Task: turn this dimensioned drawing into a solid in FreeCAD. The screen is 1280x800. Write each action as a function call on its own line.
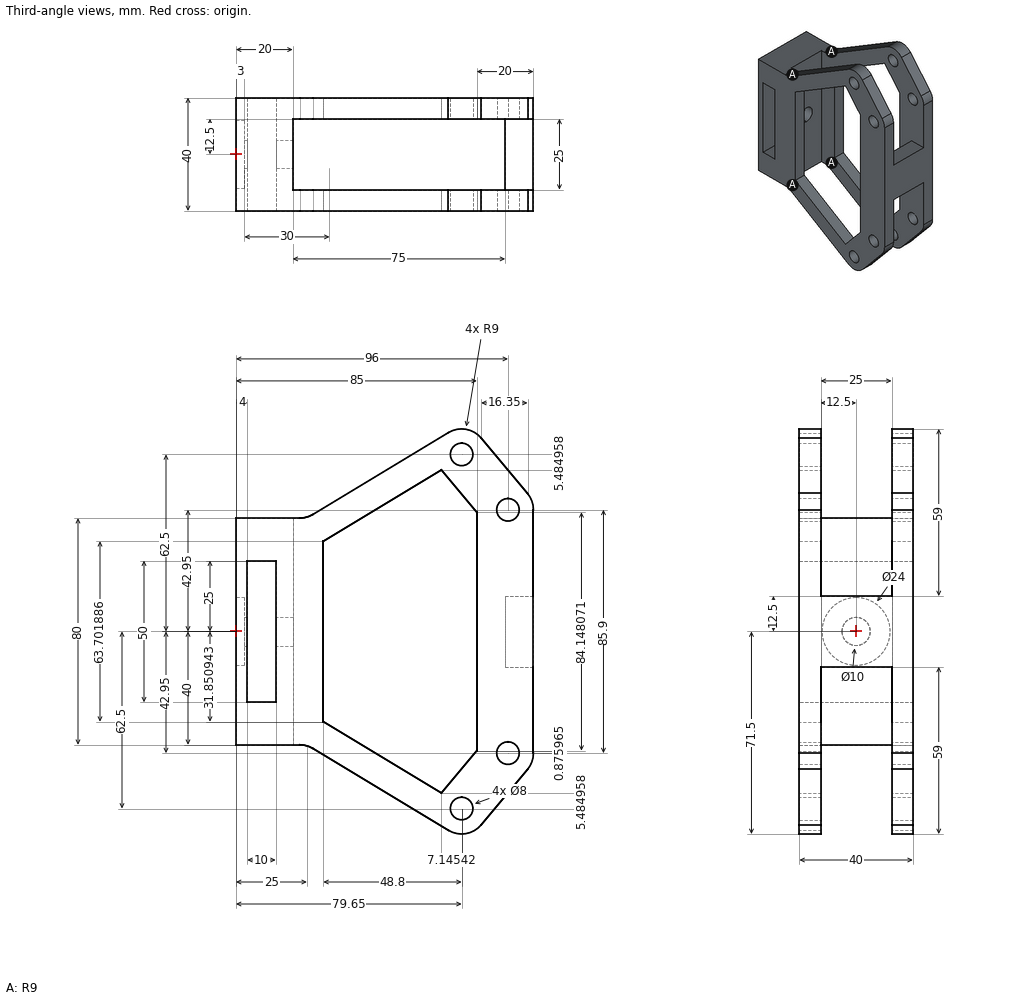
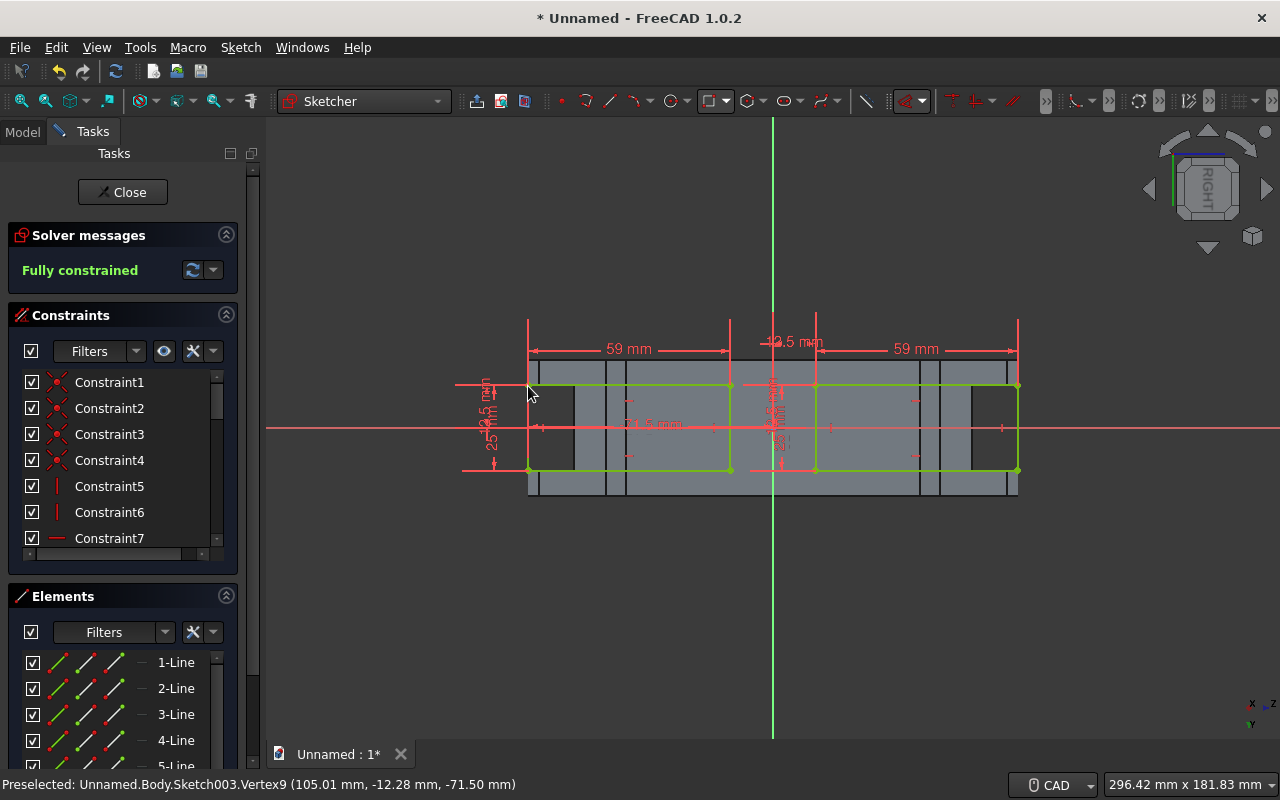
click(123, 192)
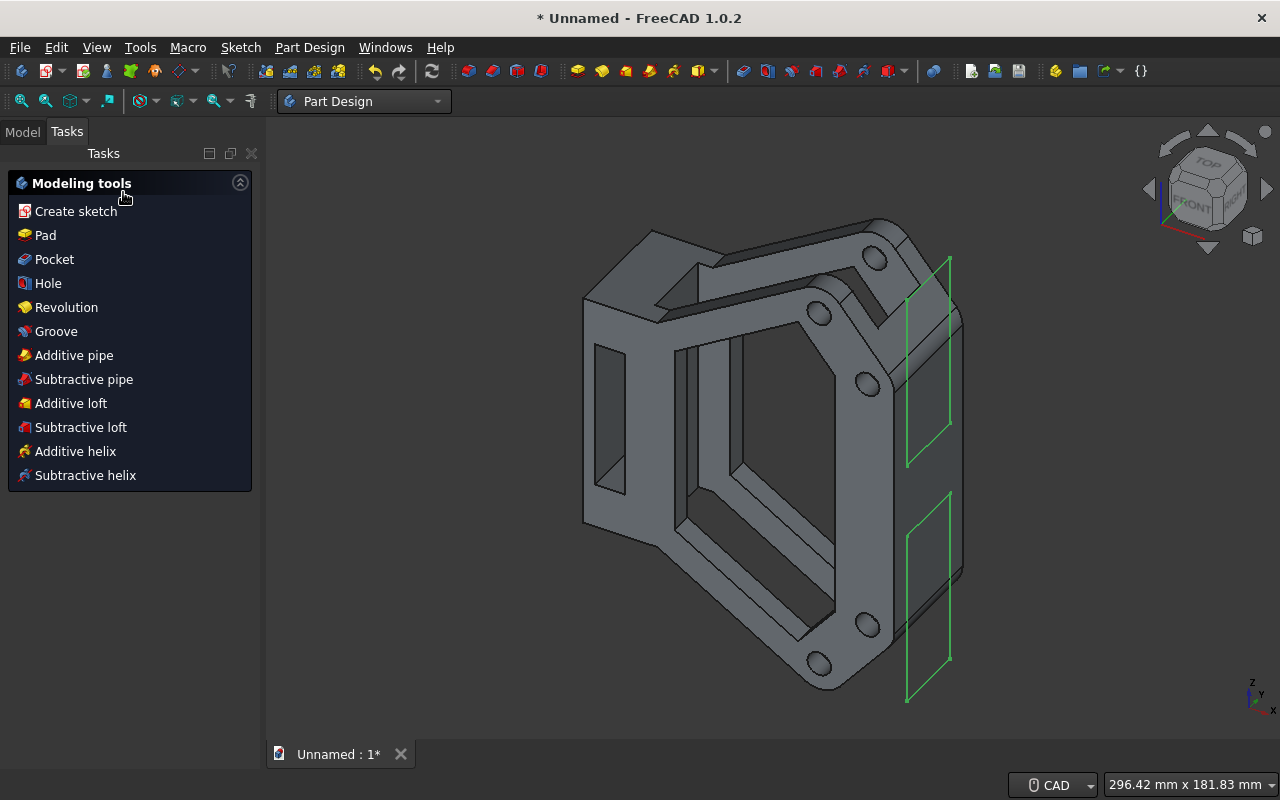
click(744, 72)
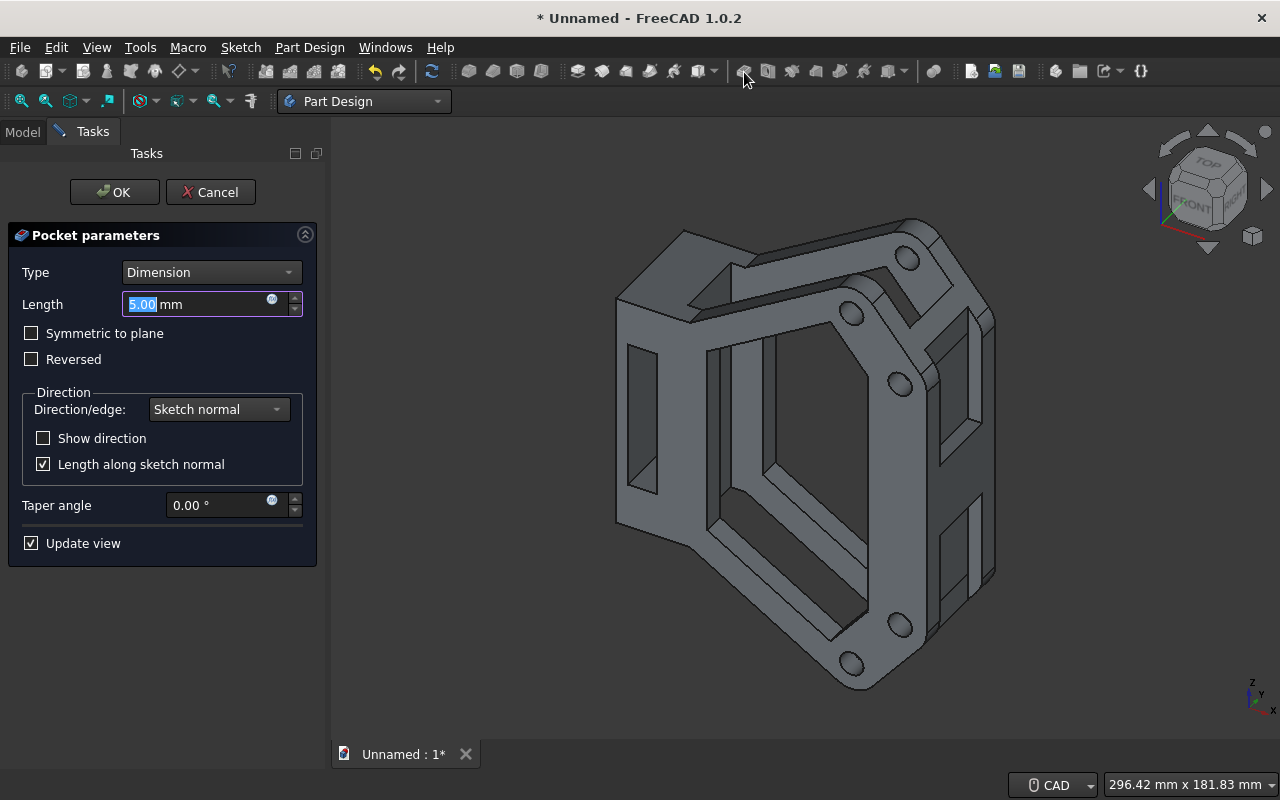
text(20)
key(Tab)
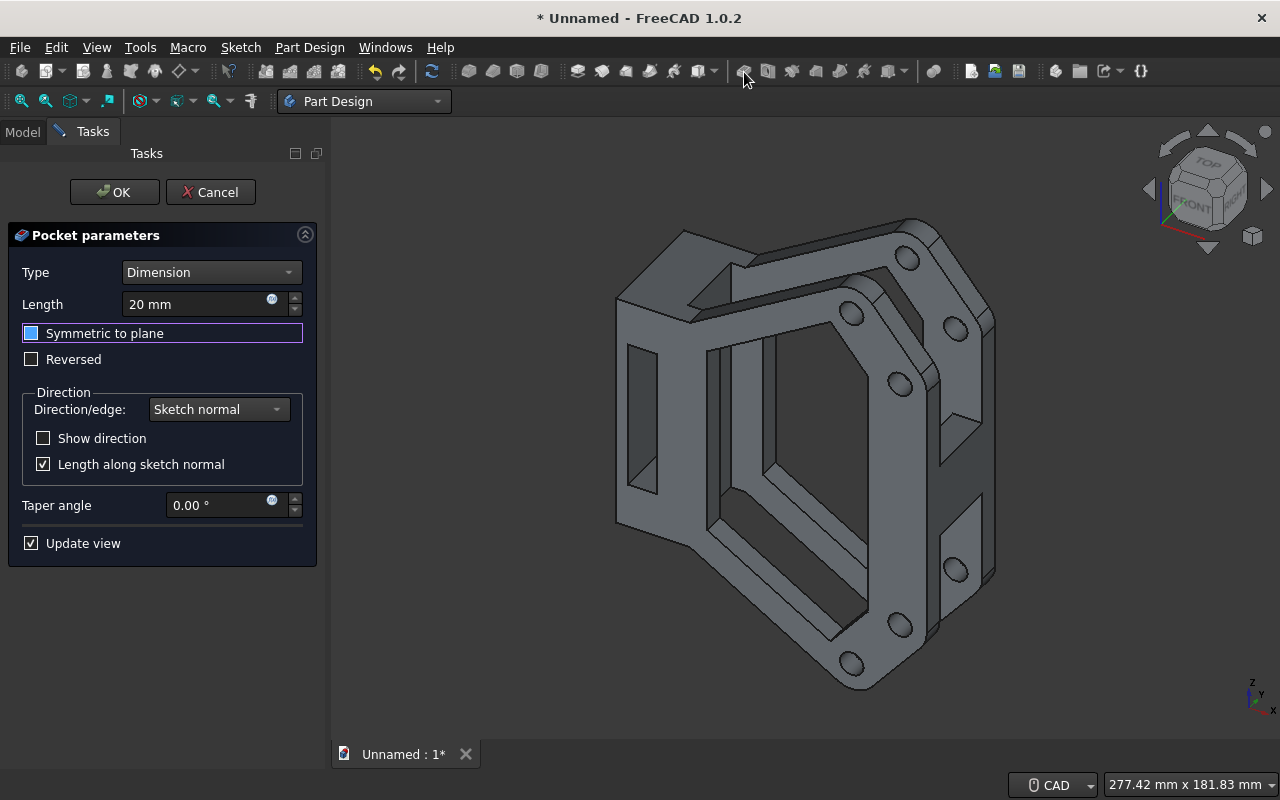
click(115, 192)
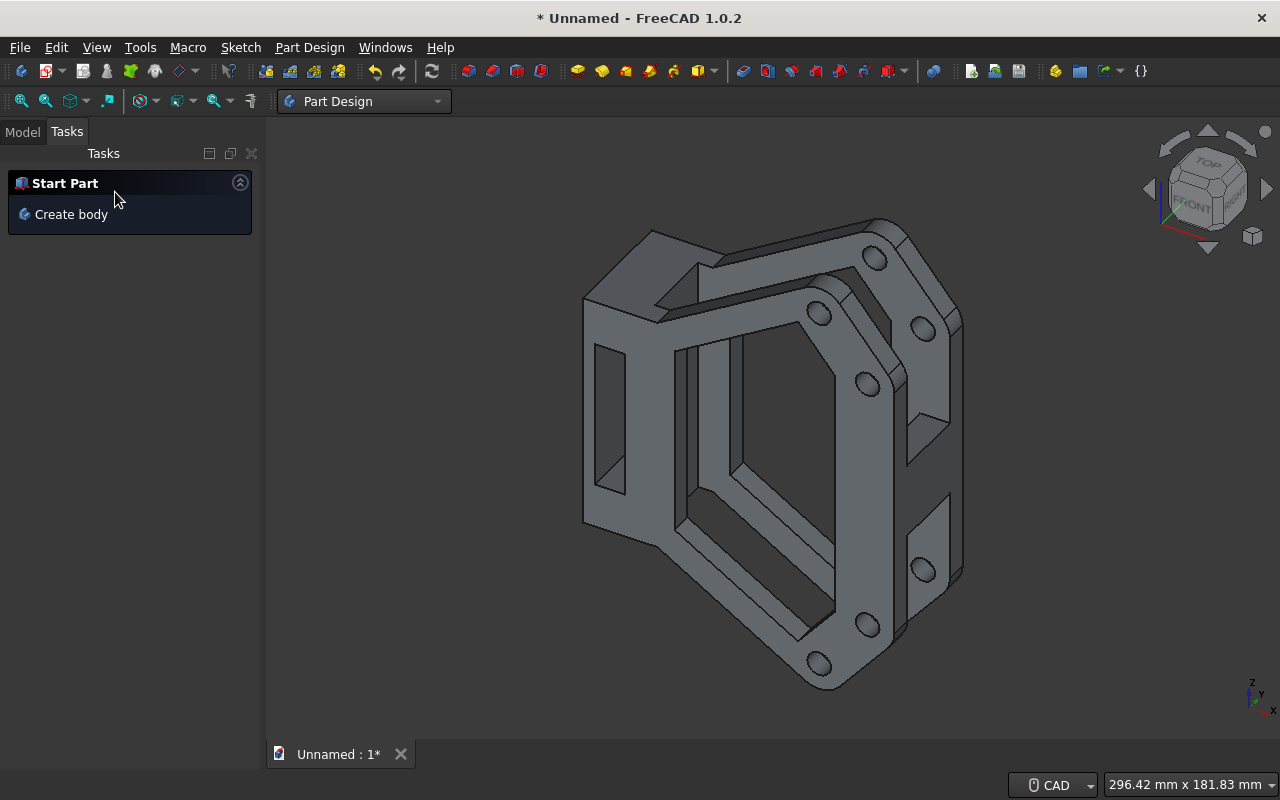
click(46, 72)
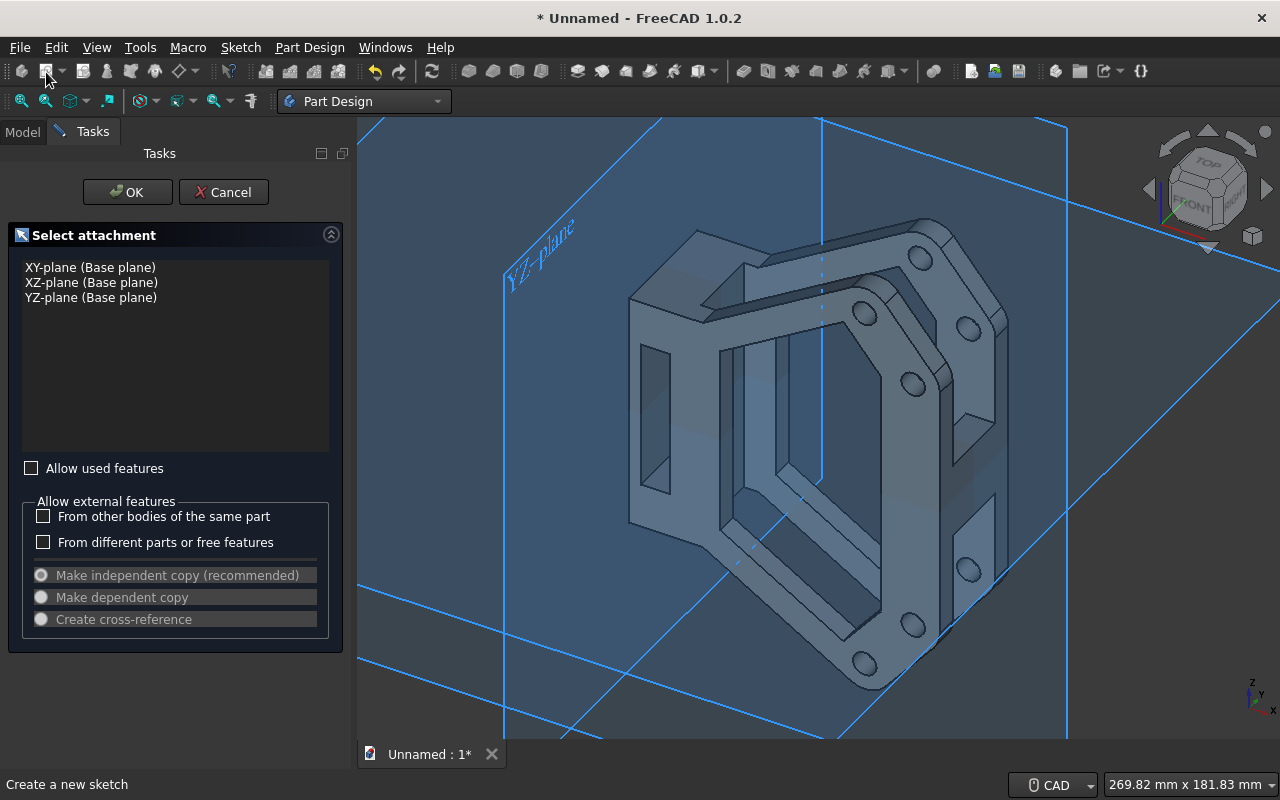
click(82, 298)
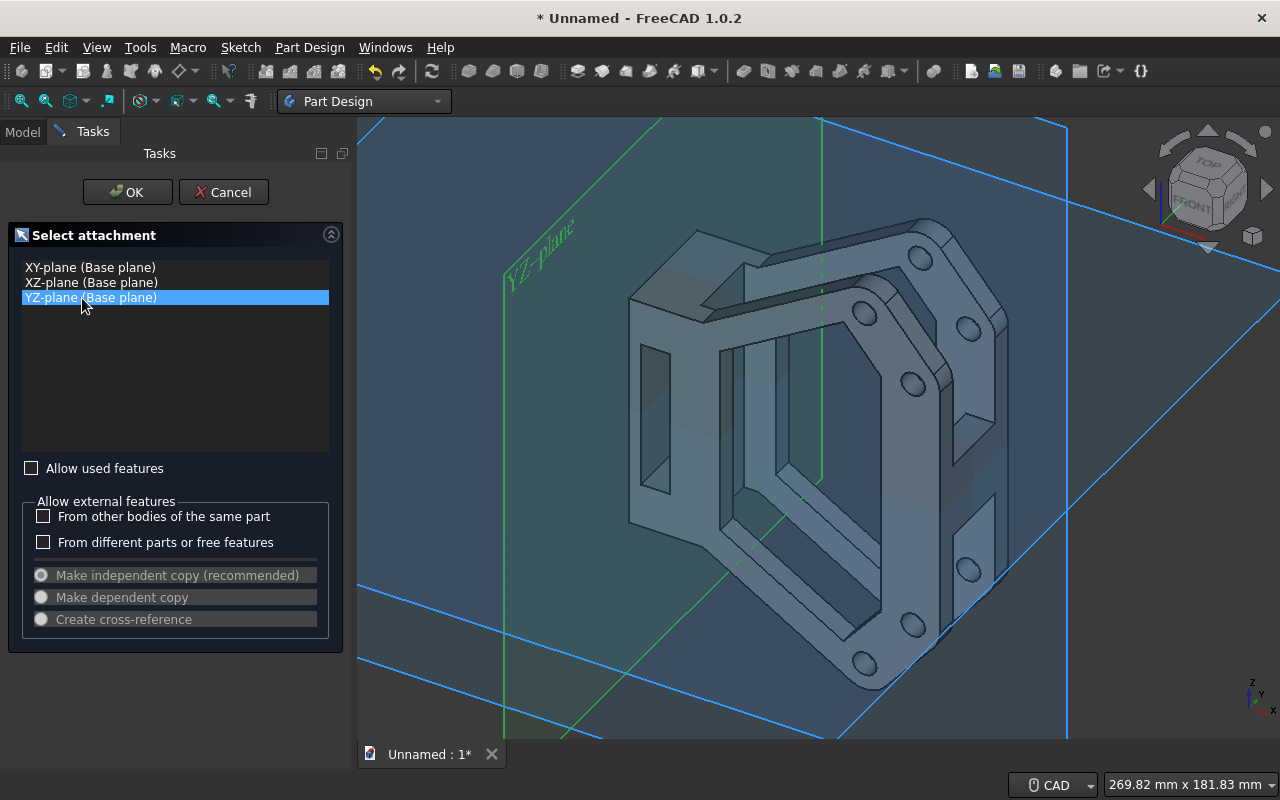
click(128, 192)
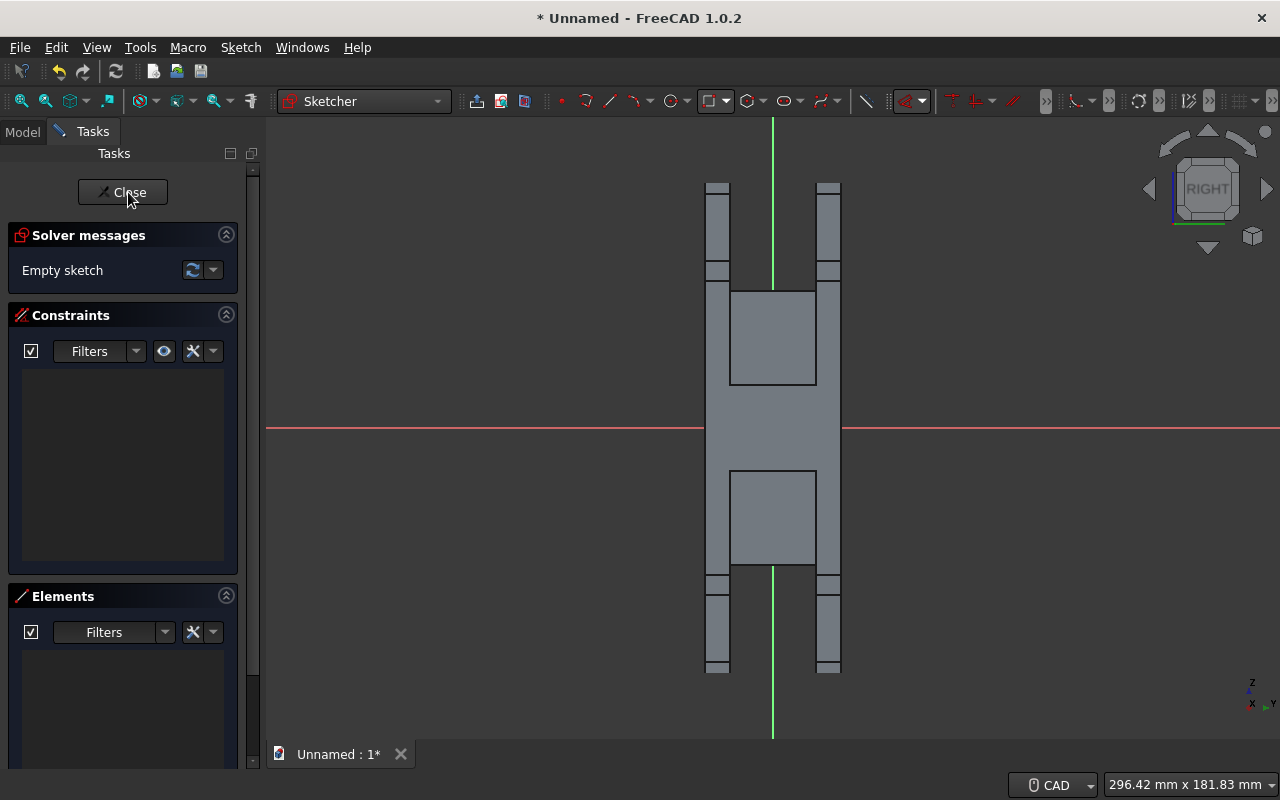
click(526, 102)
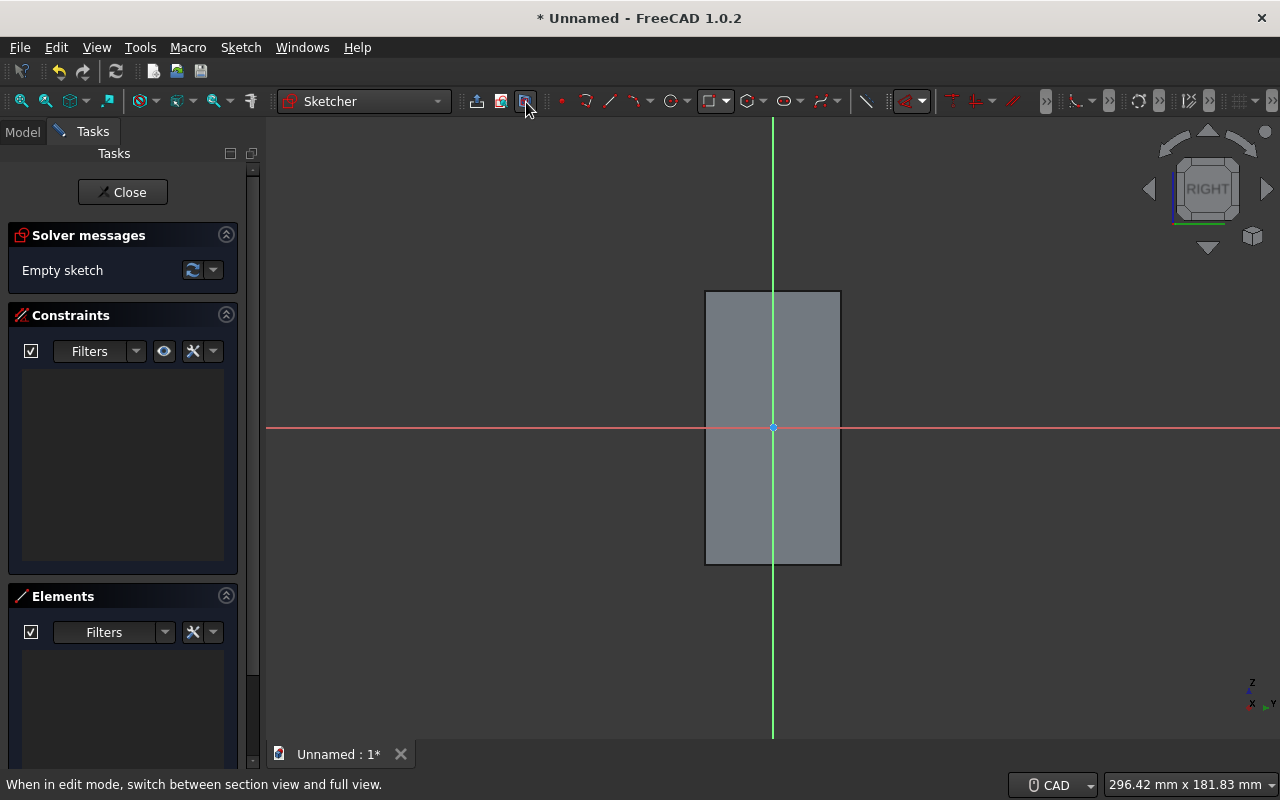
scroll(790, 428, up, 8)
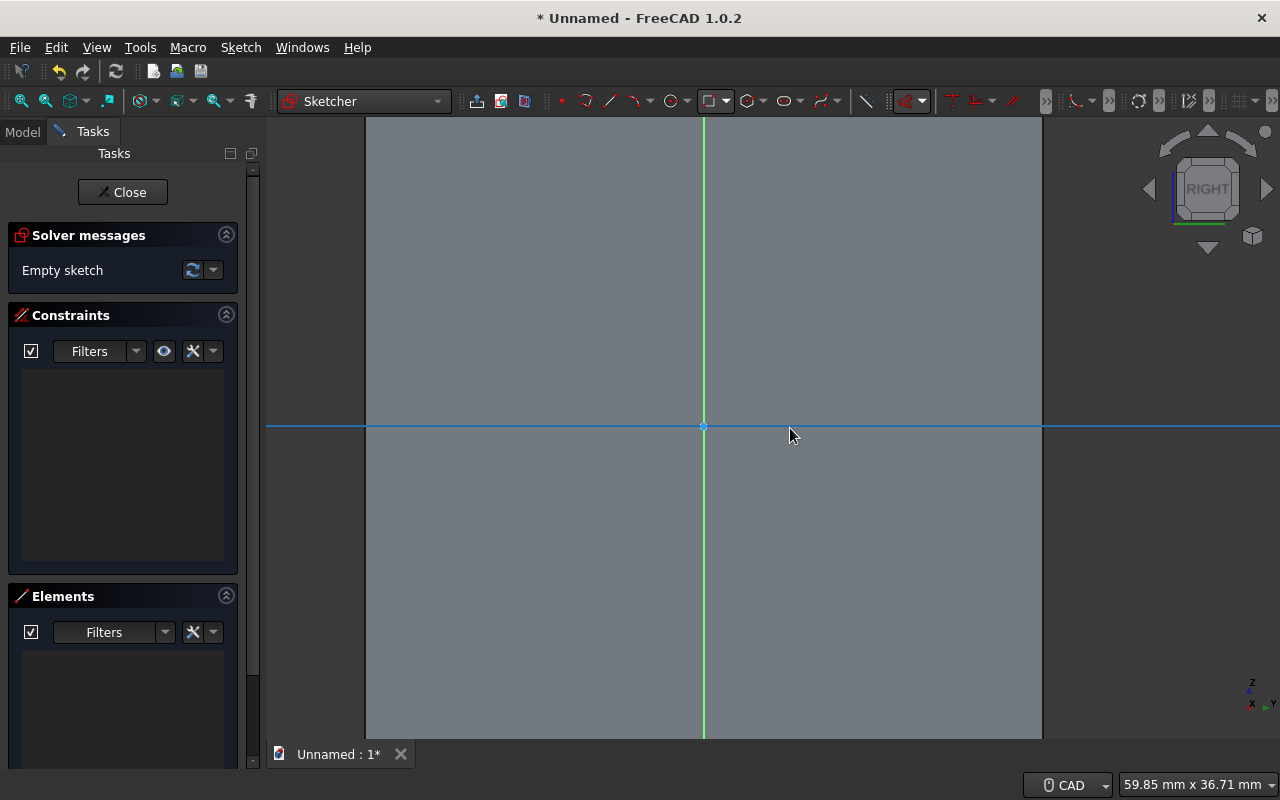
click(672, 102)